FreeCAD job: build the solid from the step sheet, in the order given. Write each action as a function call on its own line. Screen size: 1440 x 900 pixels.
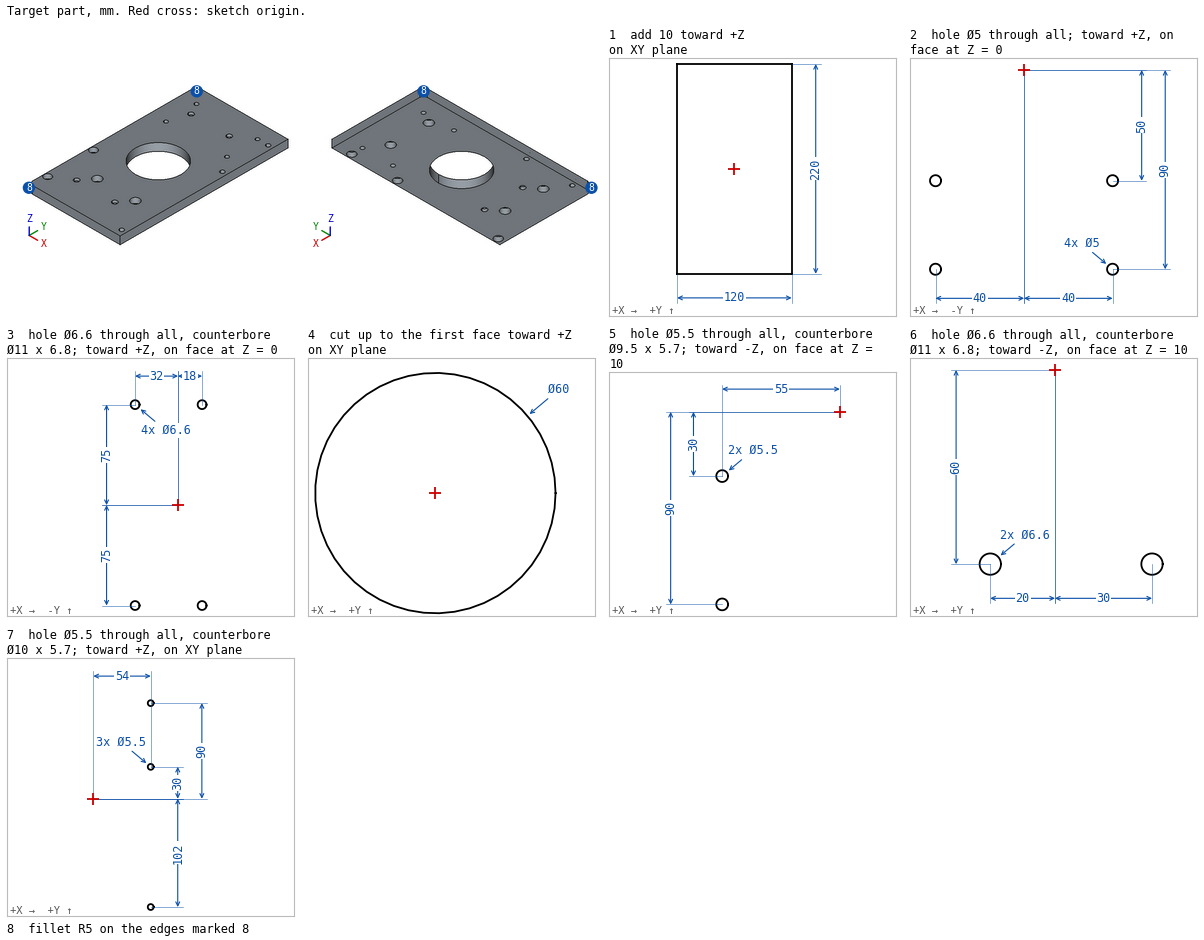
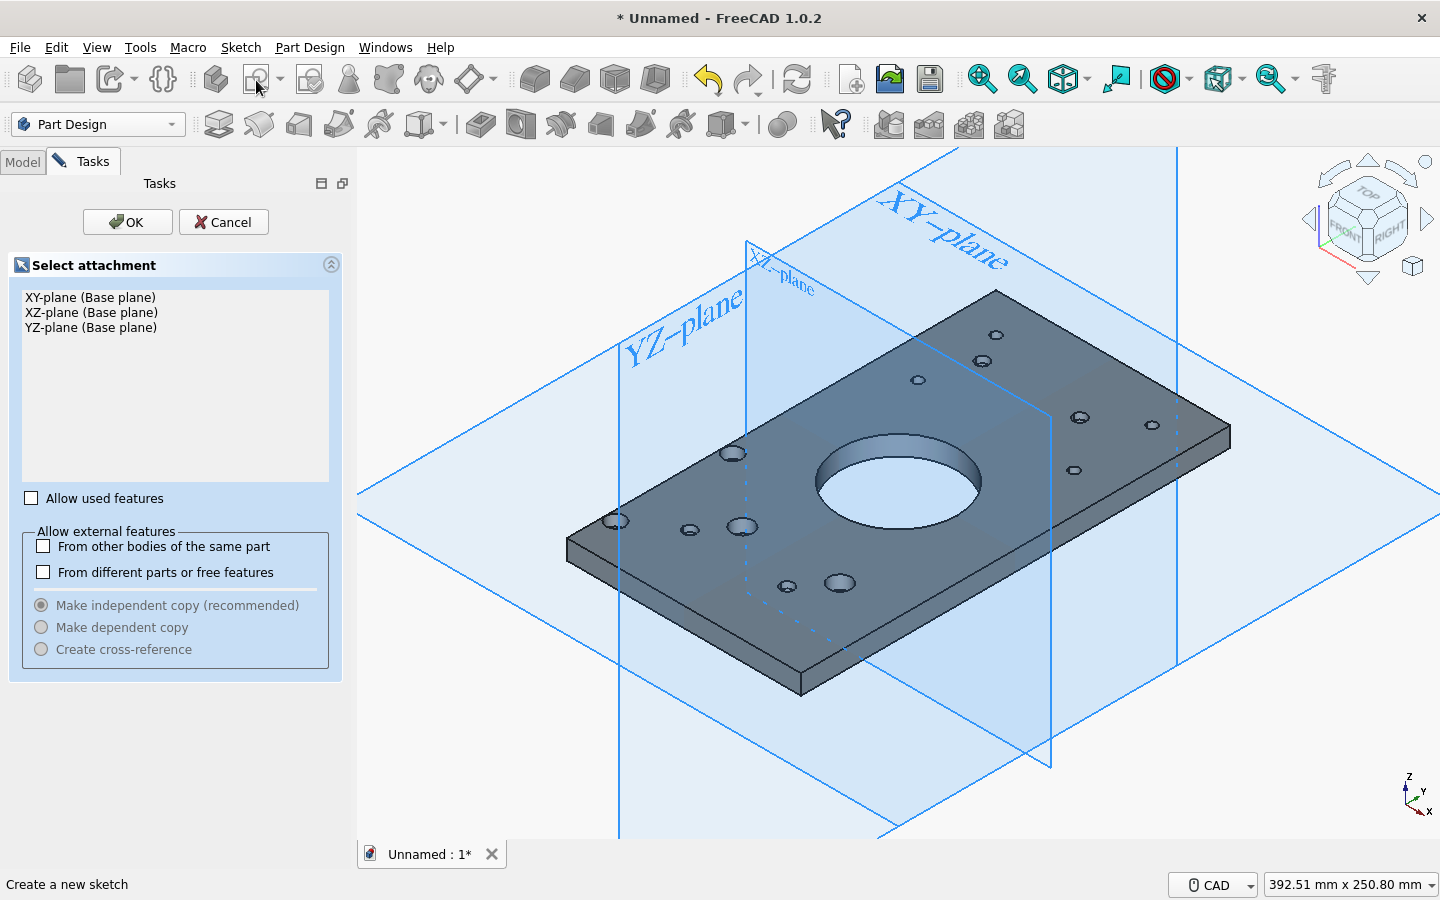
click(82, 298)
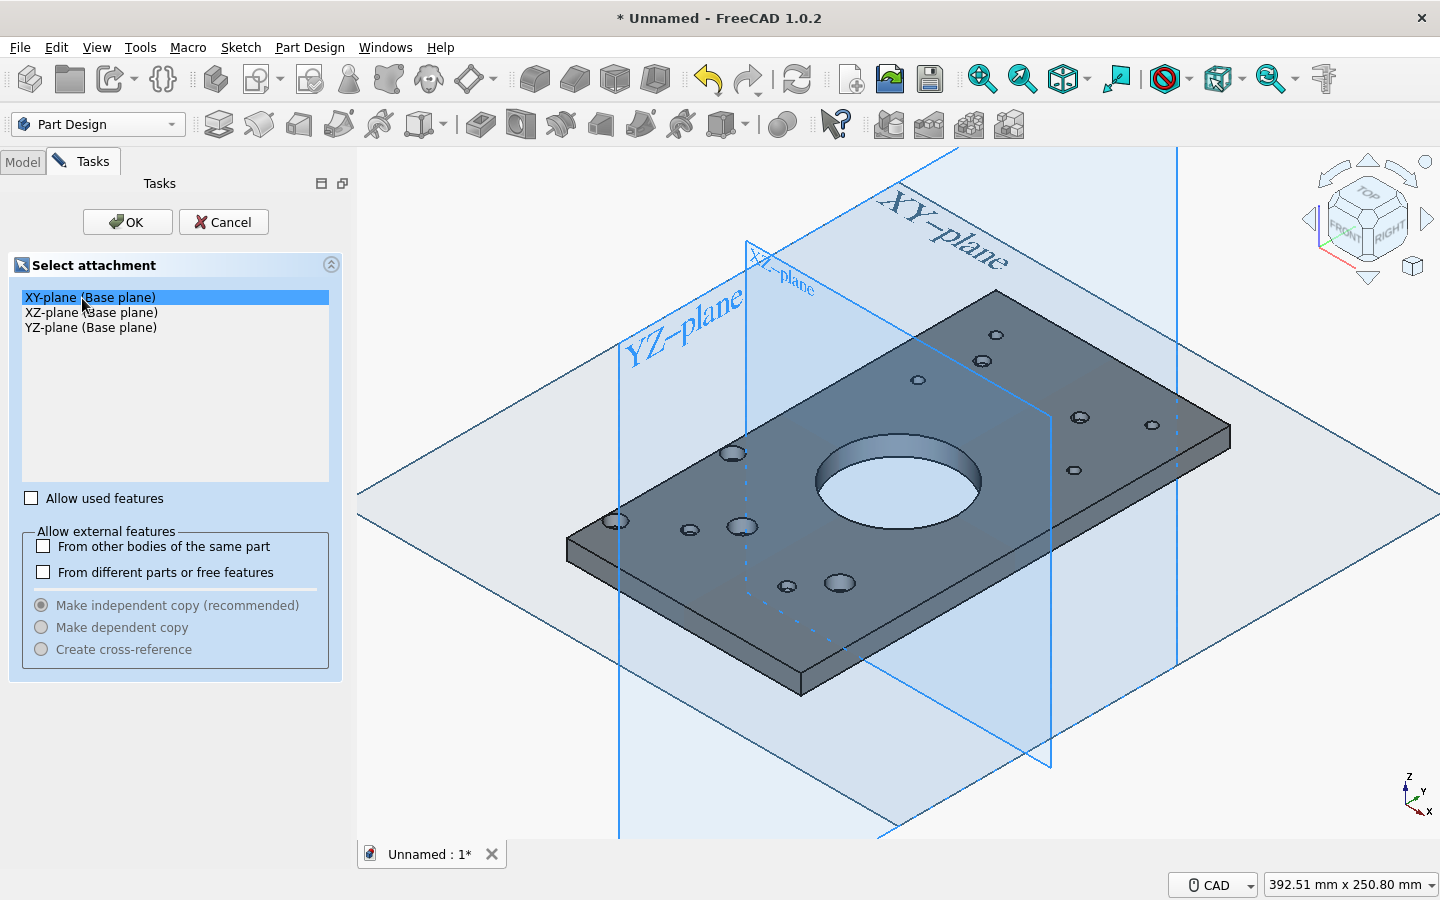
click(128, 222)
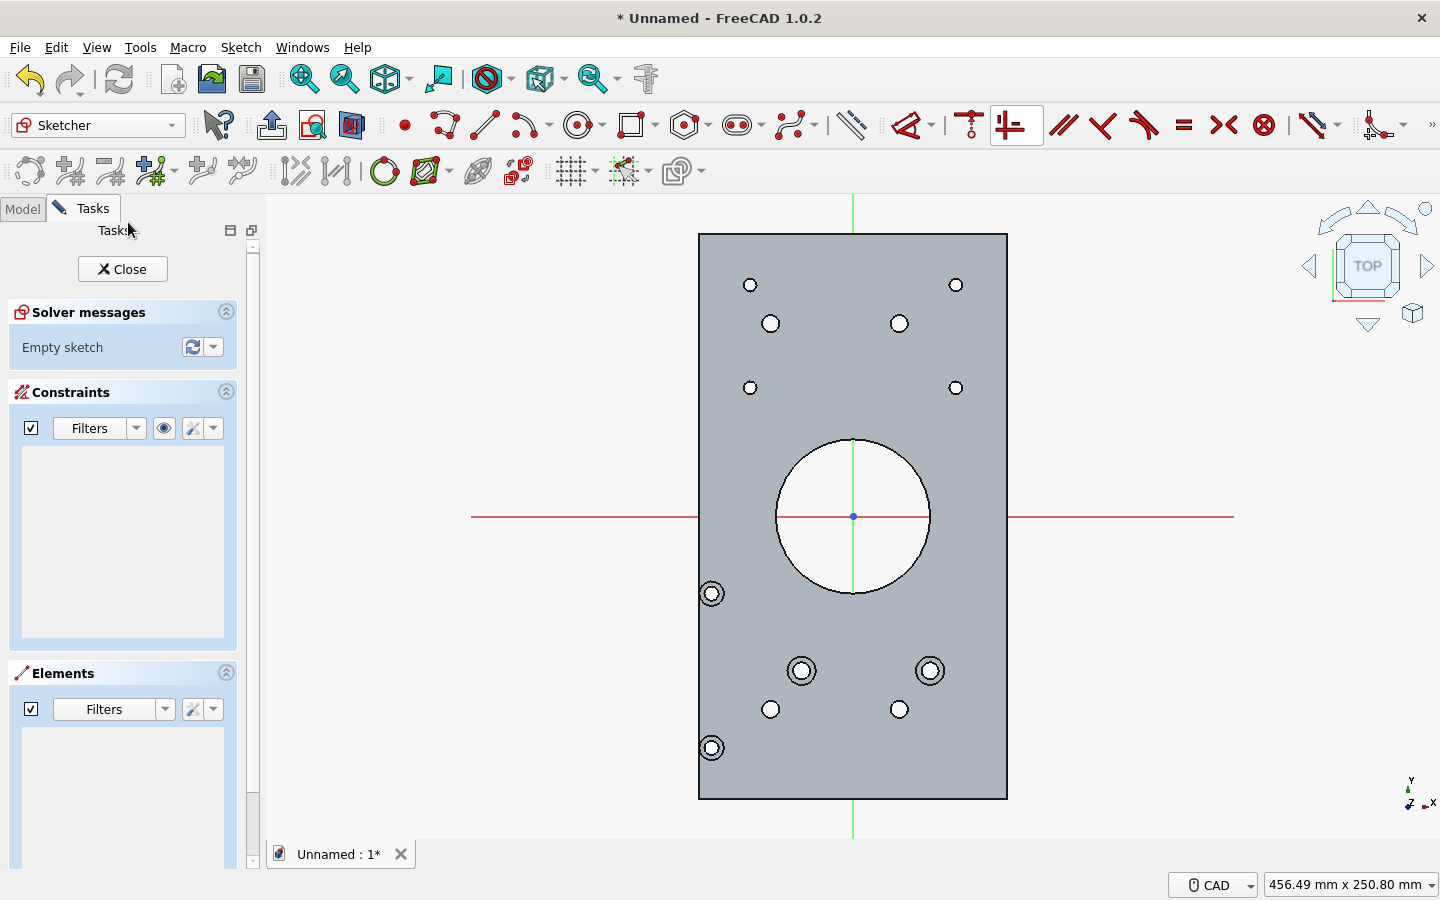
click(352, 126)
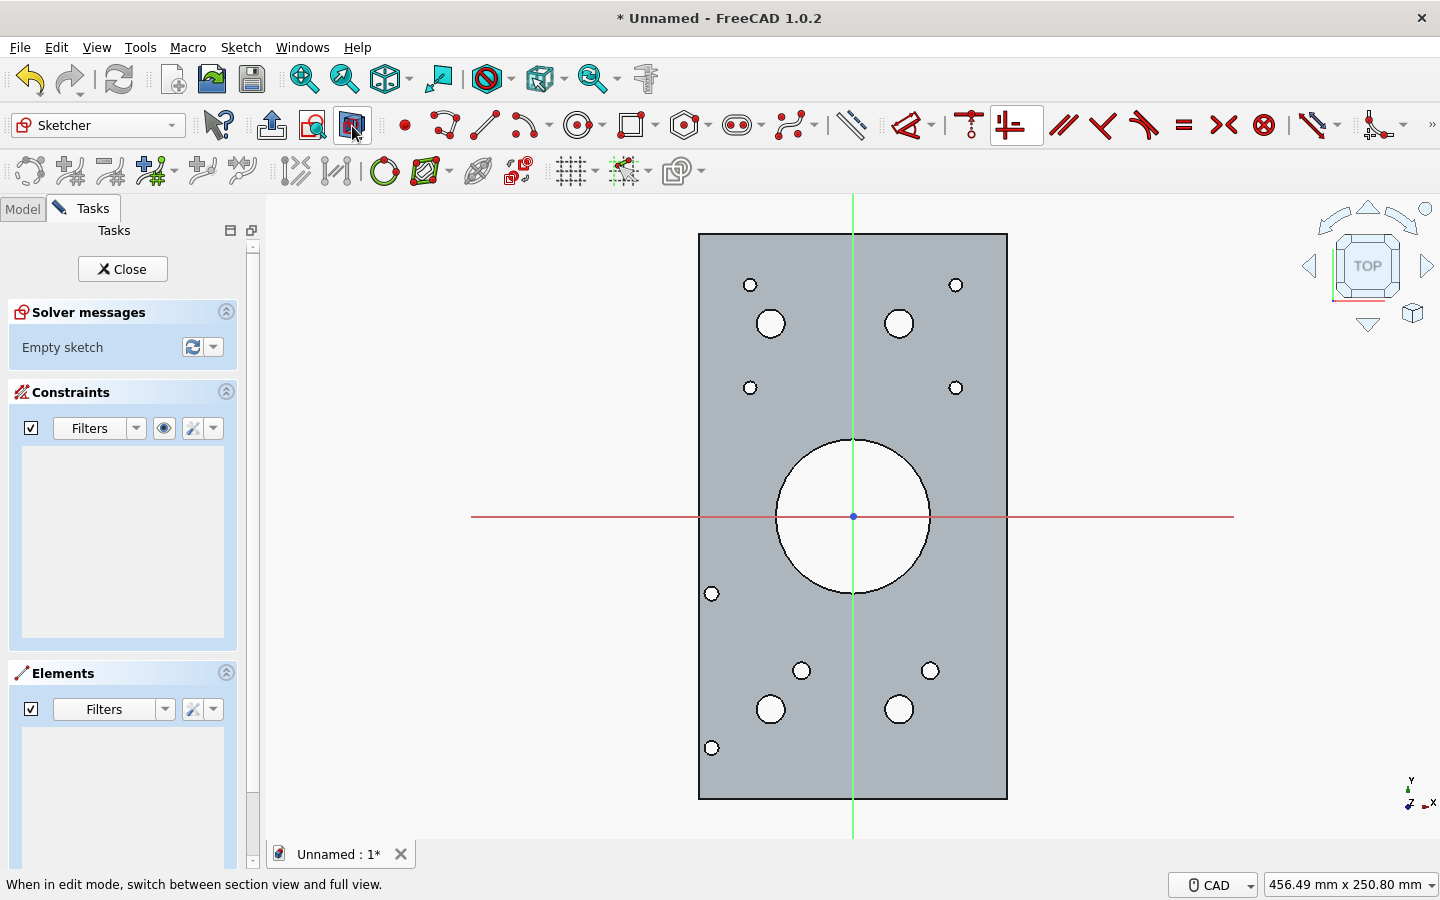
click(578, 126)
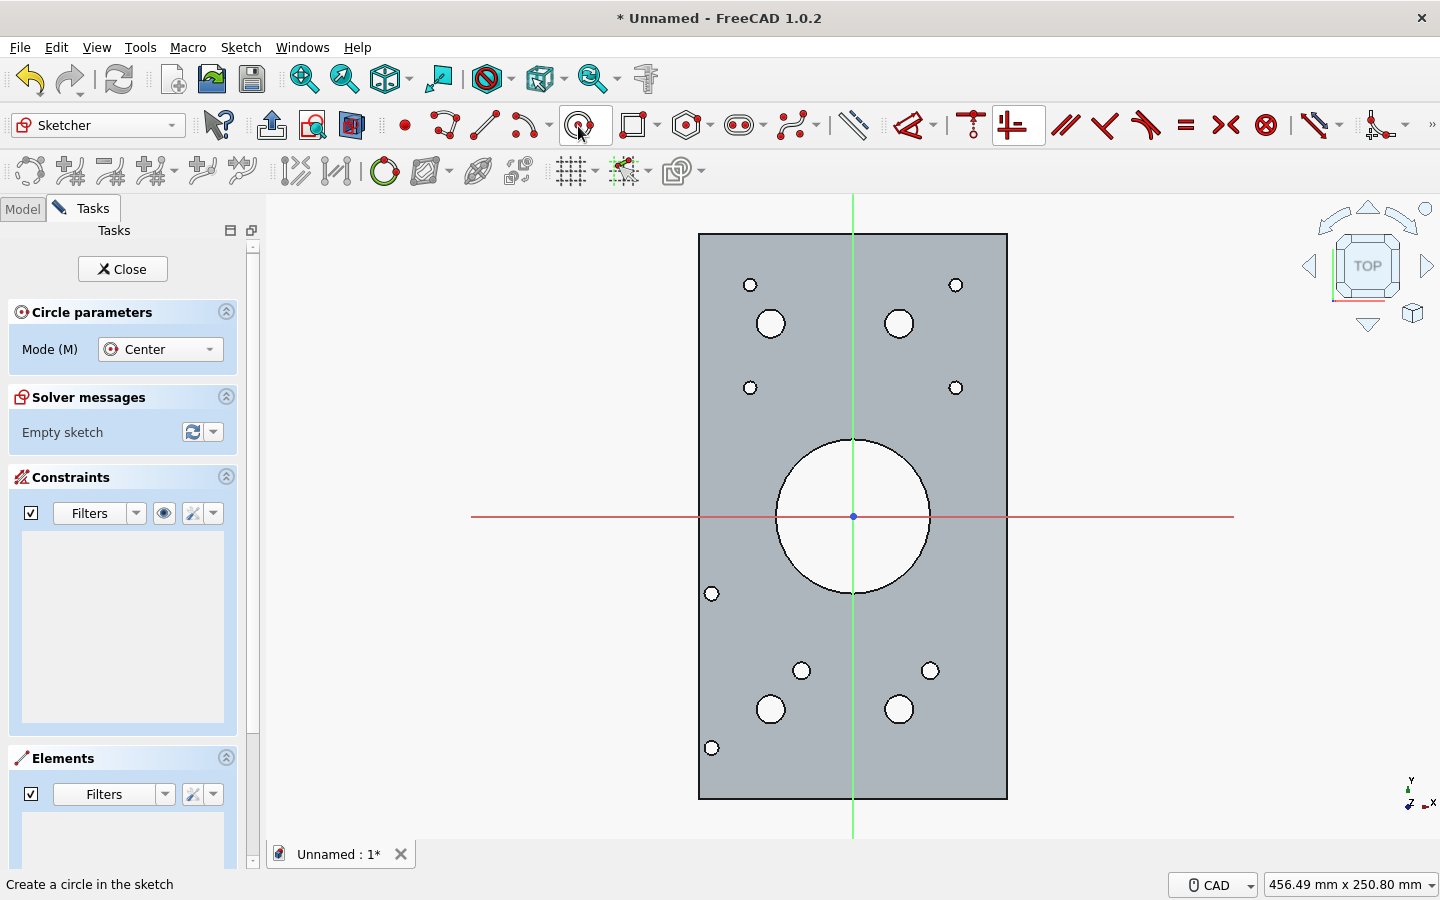
scroll(992, 439, up, 6)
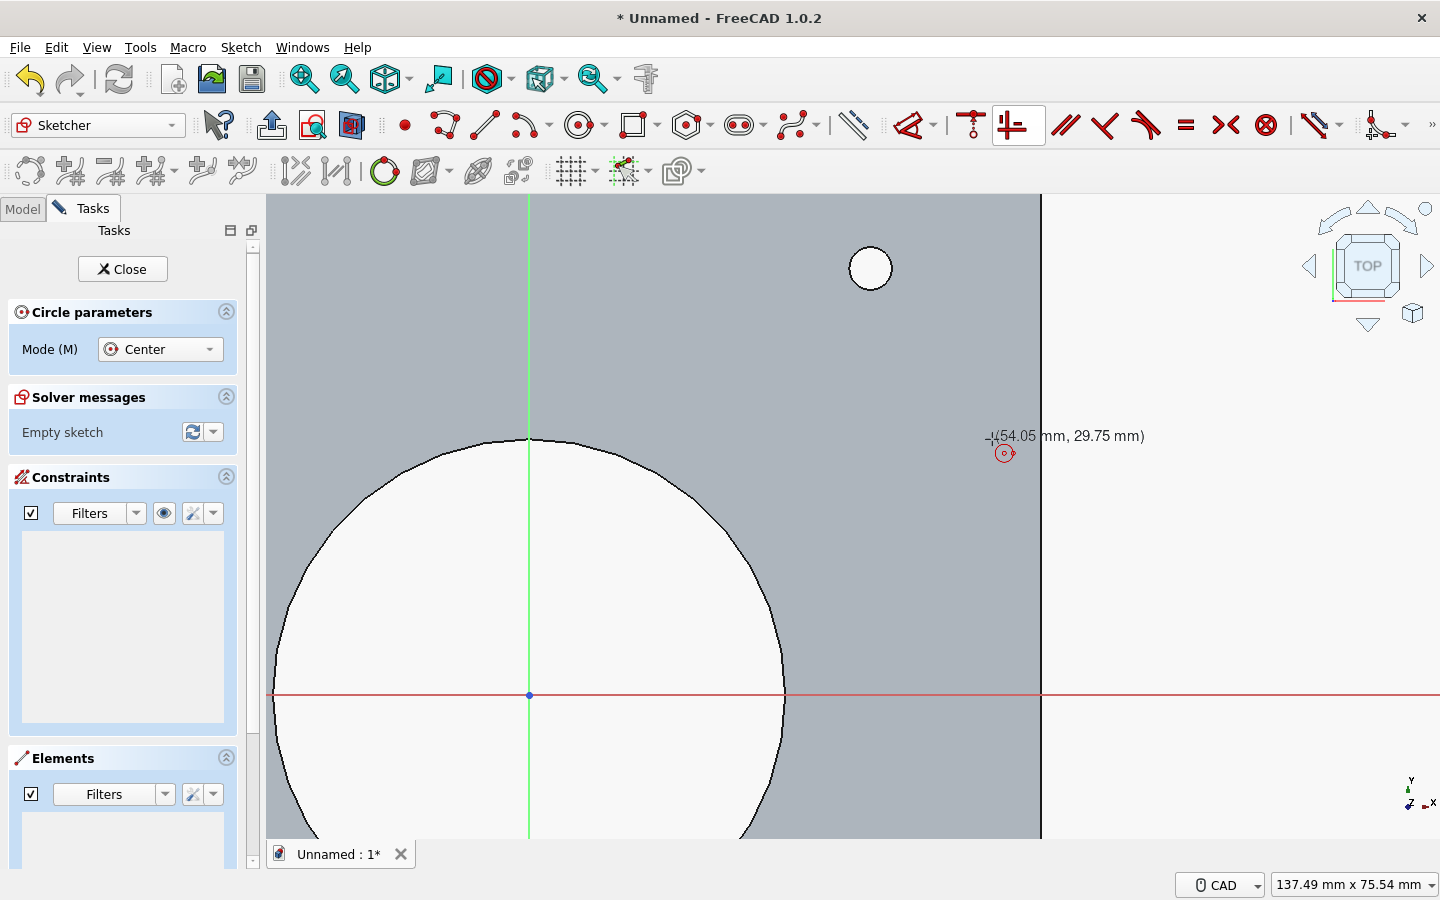
click(990, 439)
move(1007, 423)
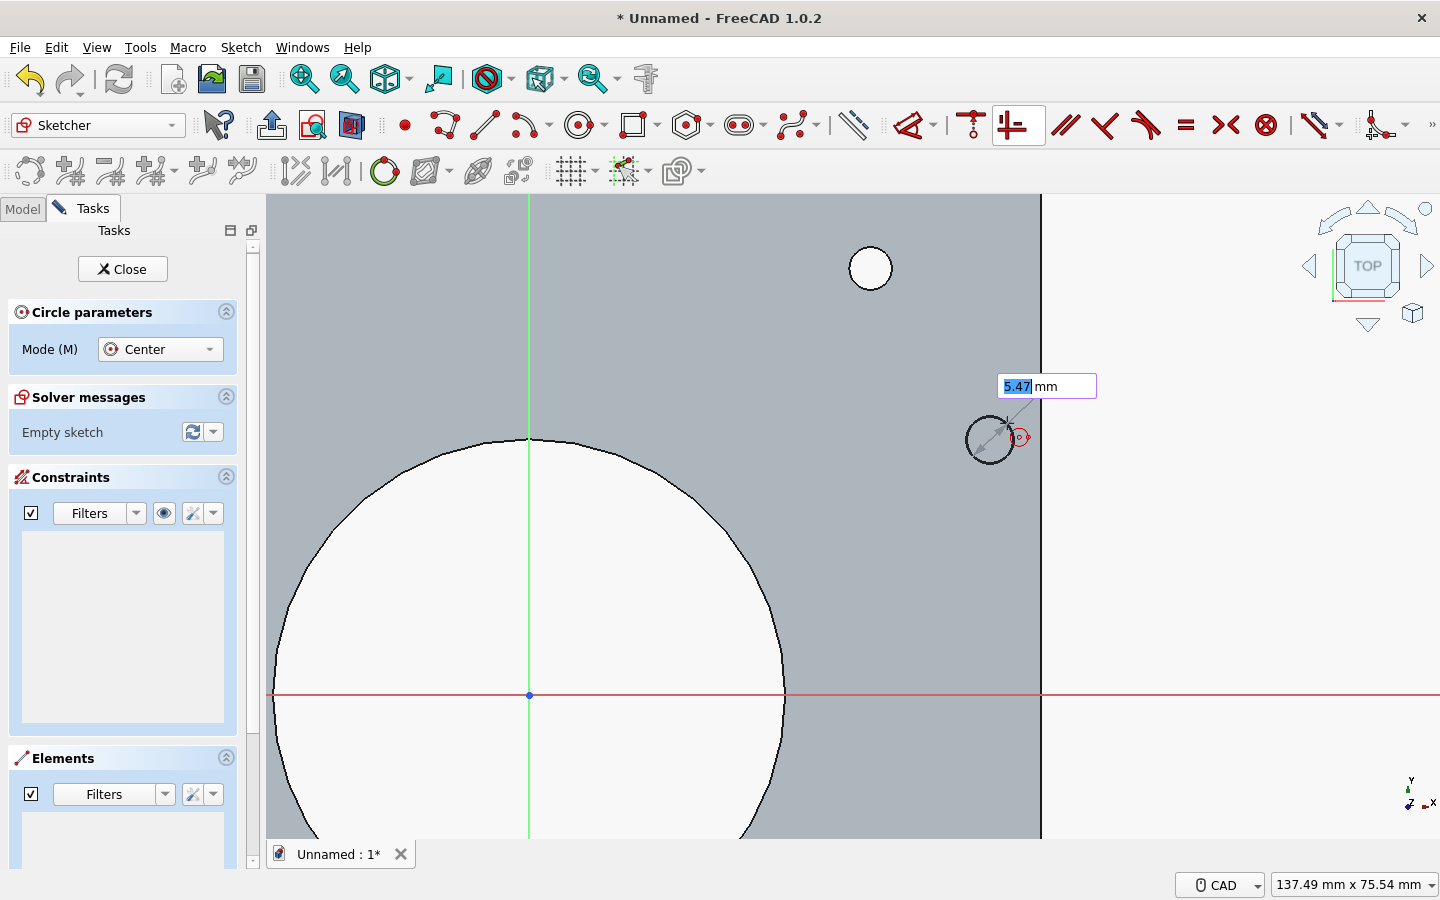
text(5.5)
key(Return)